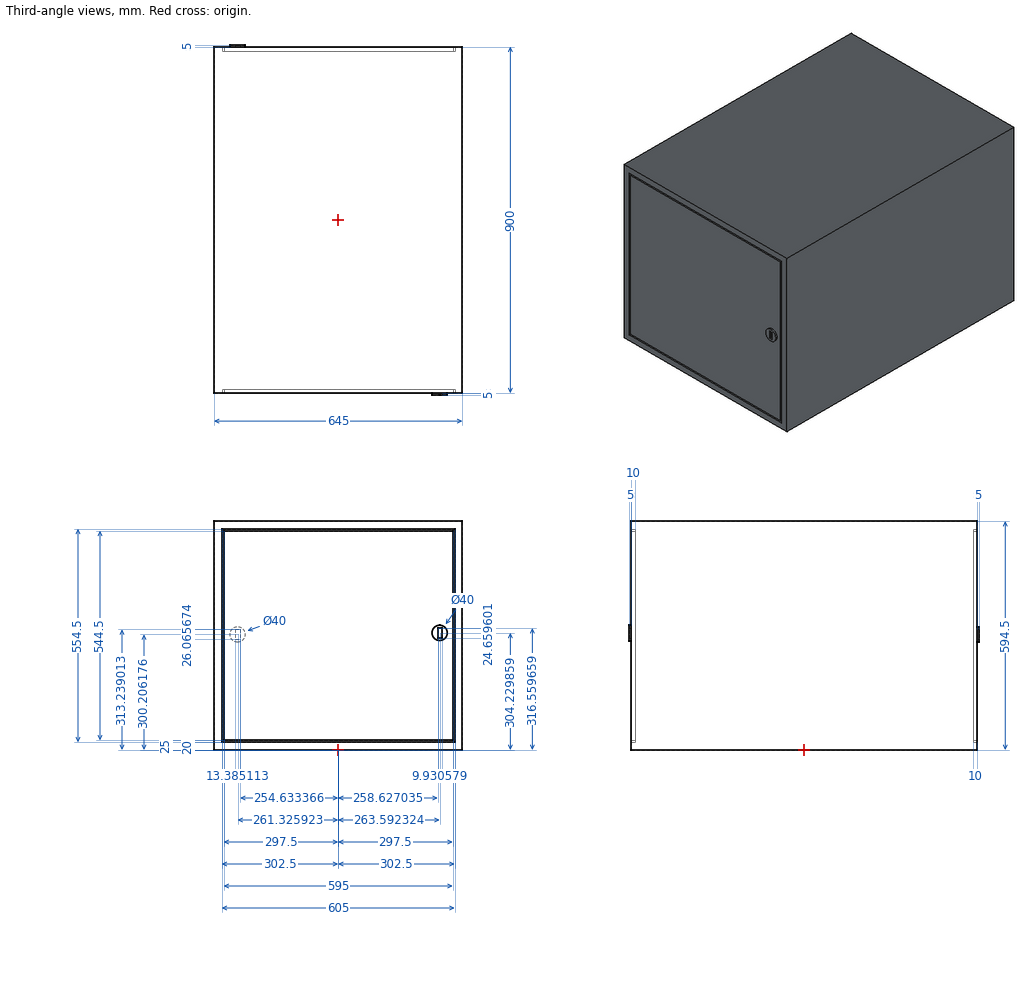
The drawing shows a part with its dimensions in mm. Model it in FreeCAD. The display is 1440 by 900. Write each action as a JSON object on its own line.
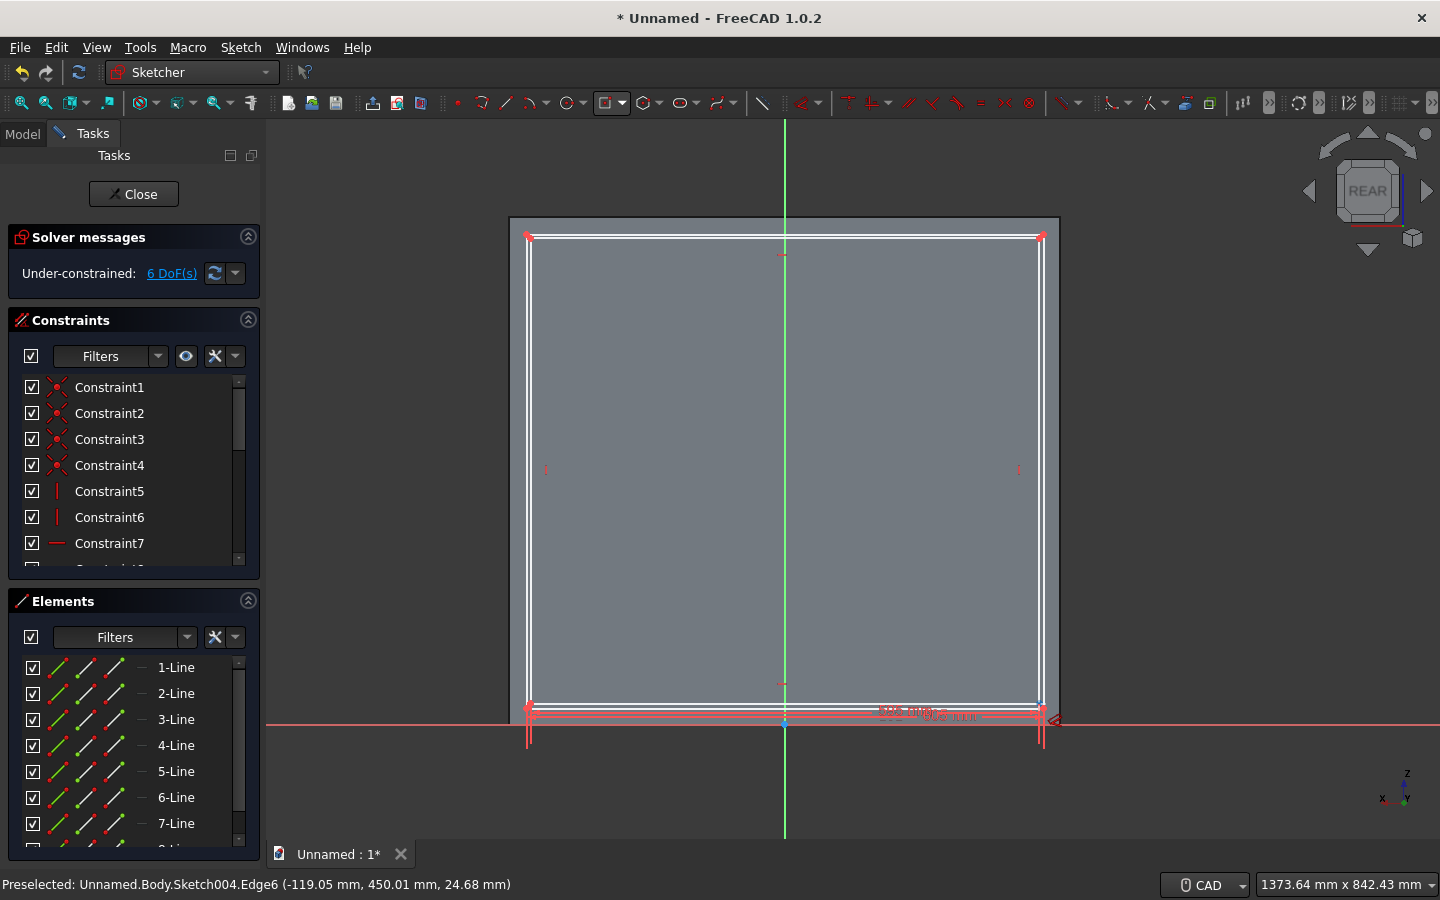
{"action": "scroll", "coordinate": [527, 709], "scroll_direction": "up", "scroll_amount": 5}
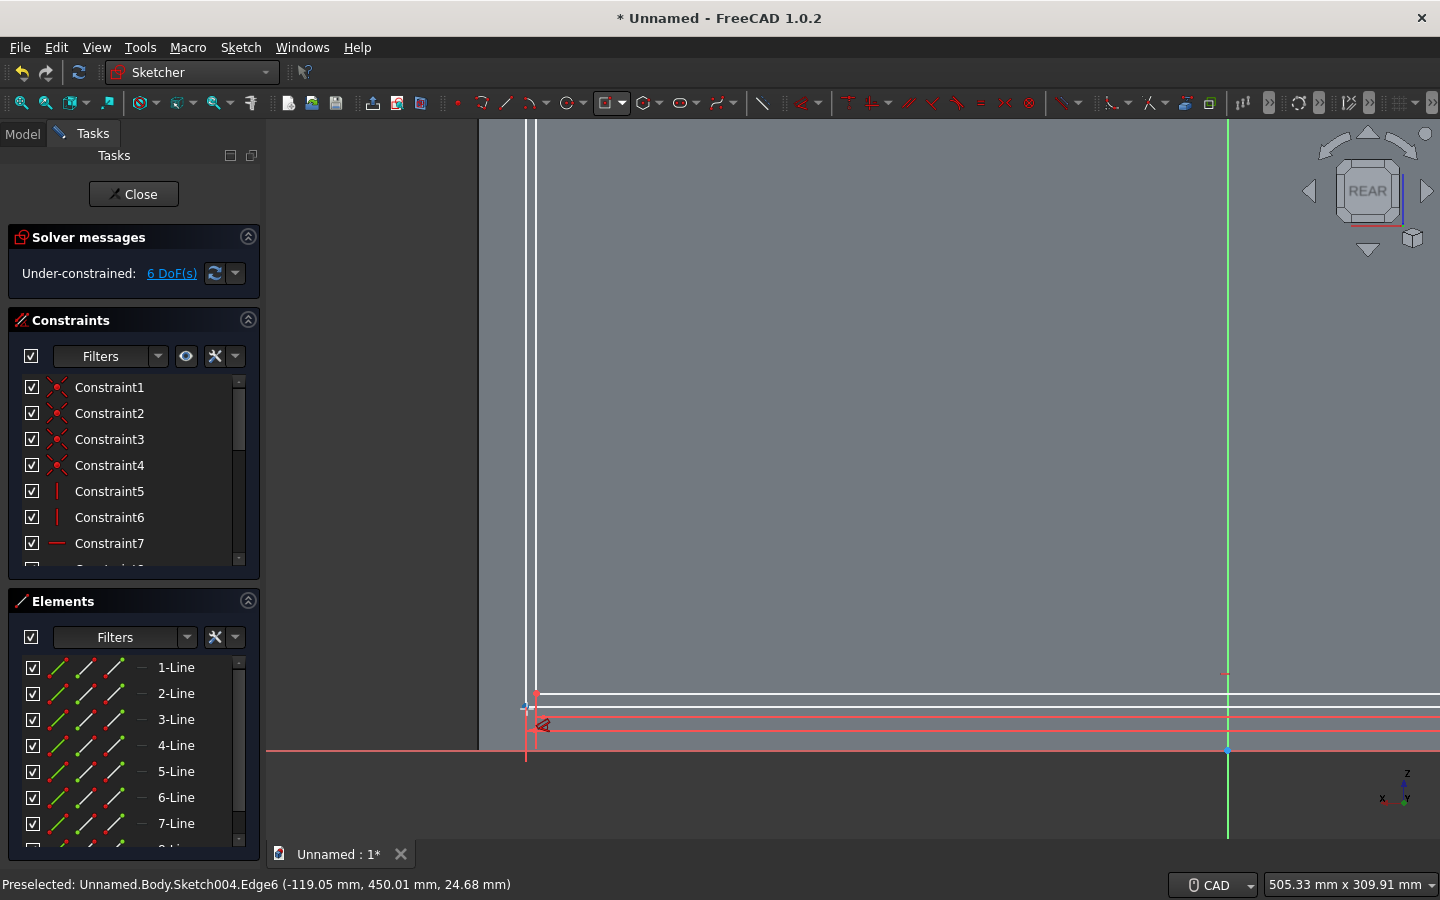
{"action": "left_click", "coordinate": [526, 707]}
{"action": "left_click", "coordinate": [492, 729]}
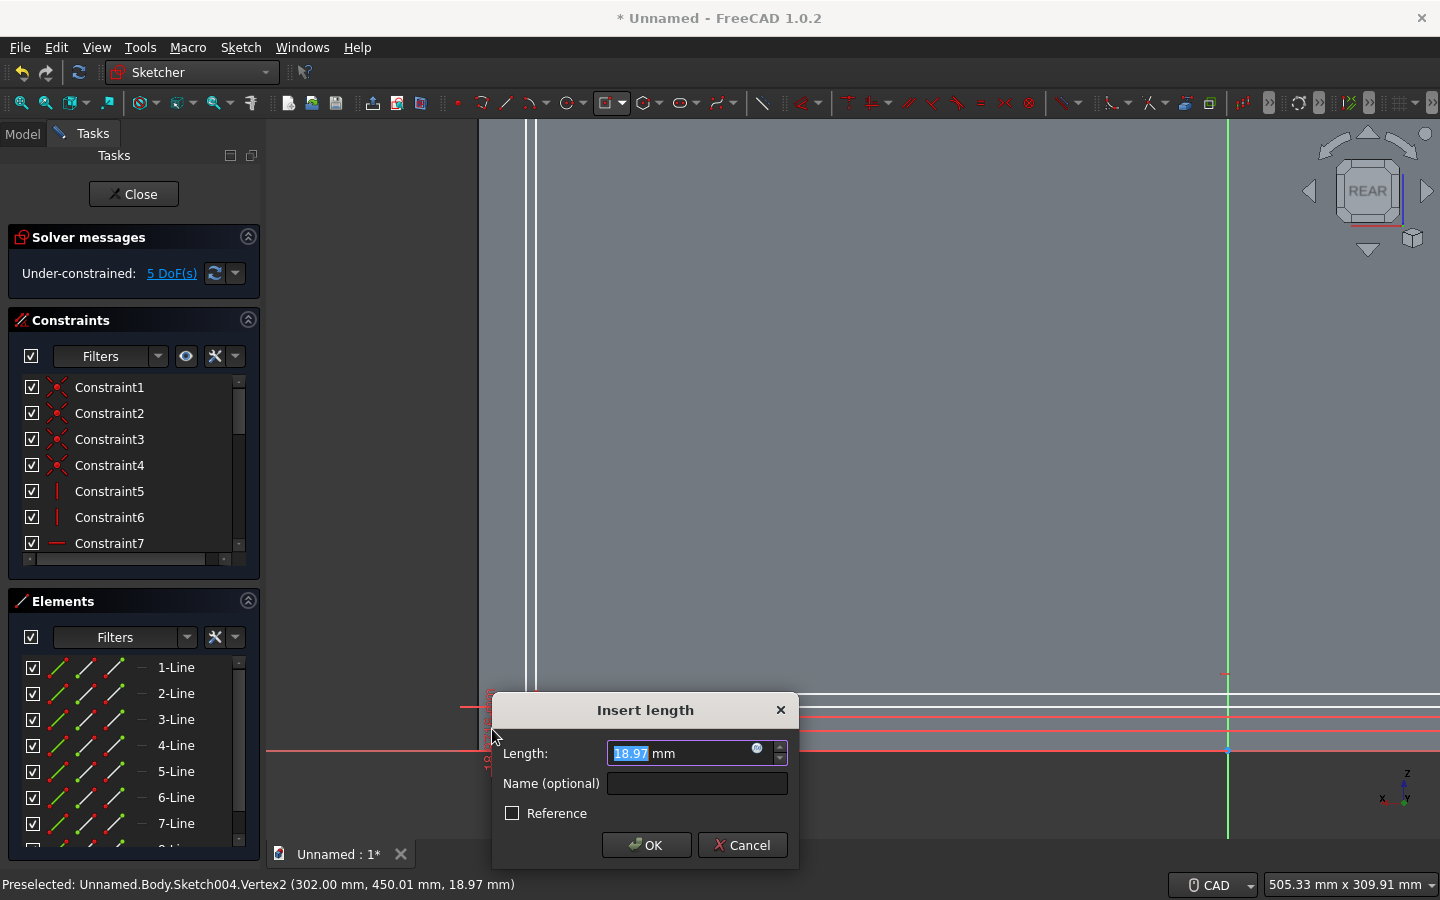
{"action": "type", "text": "20"}
{"action": "key", "text": "Return"}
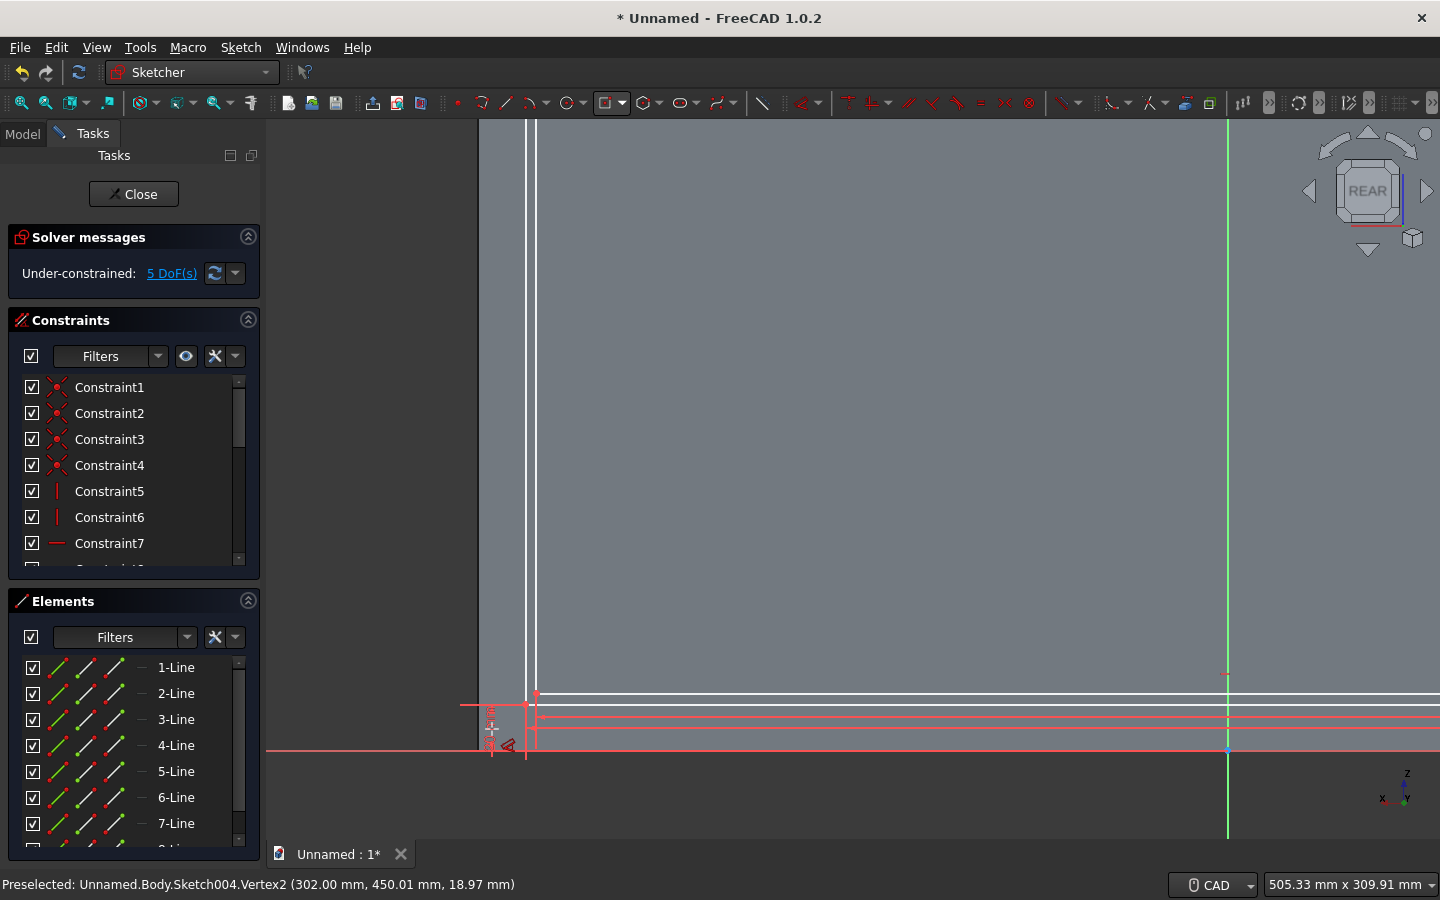
{"action": "left_click", "coordinate": [536, 694]}
{"action": "left_click", "coordinate": [502, 702]}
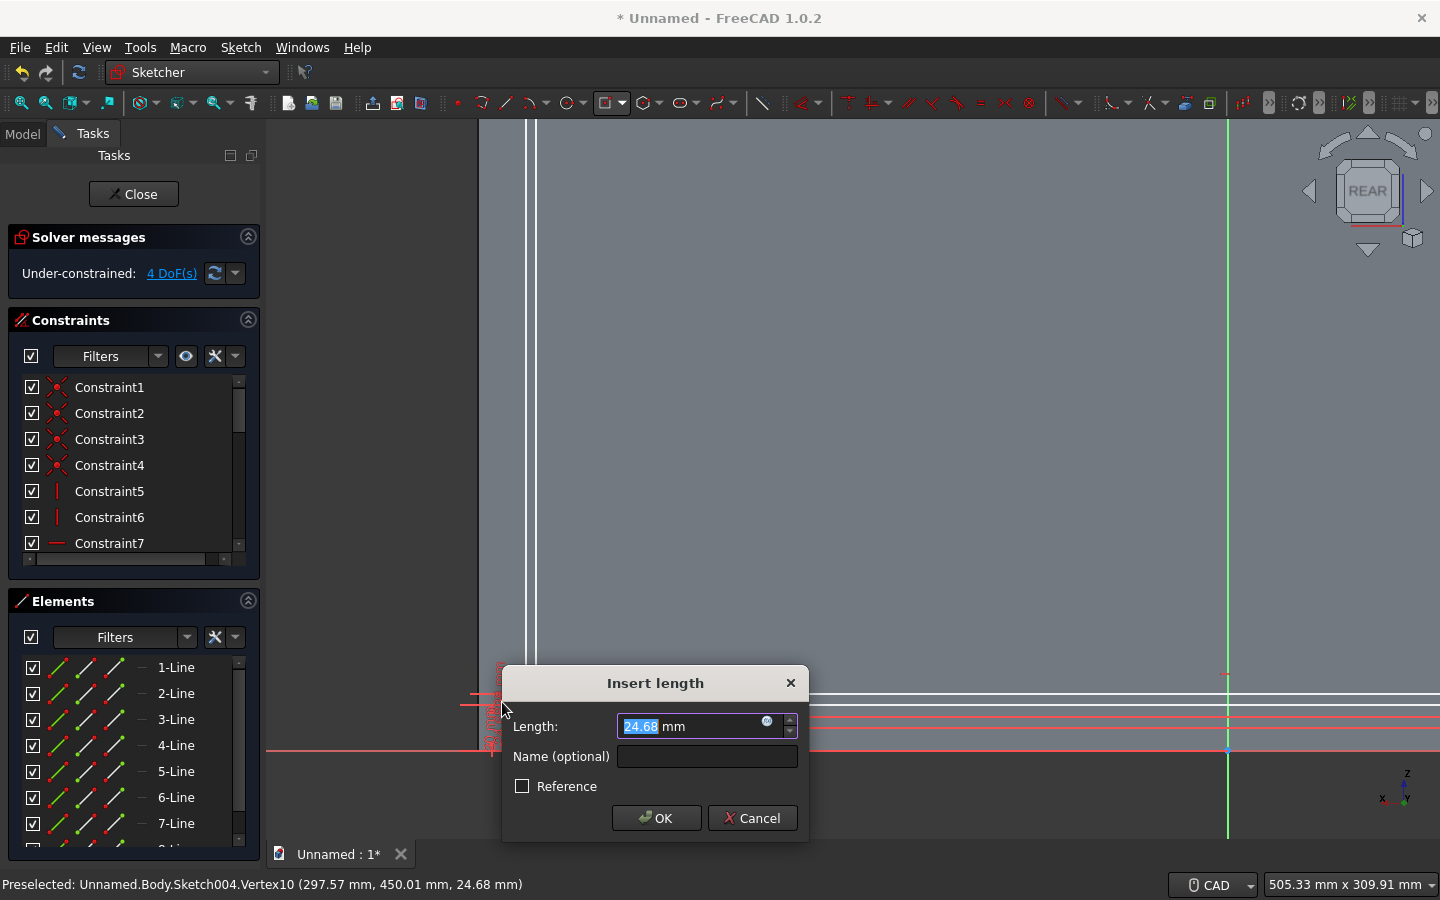
{"action": "type", "text": "25"}
{"action": "key", "text": "Return"}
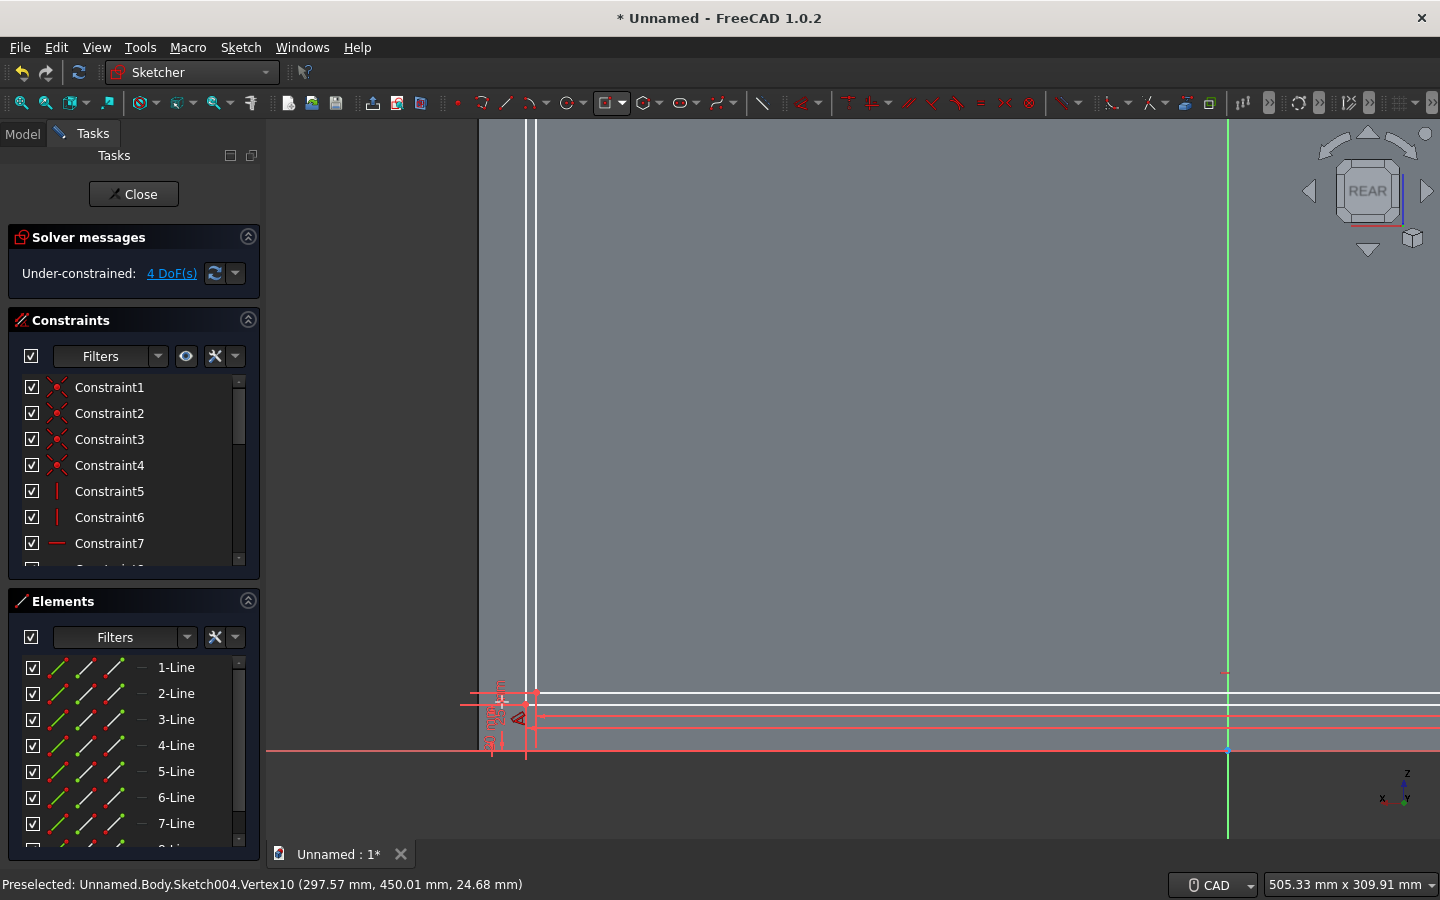
{"action": "scroll", "coordinate": [526, 319], "scroll_direction": "up", "scroll_amount": 2}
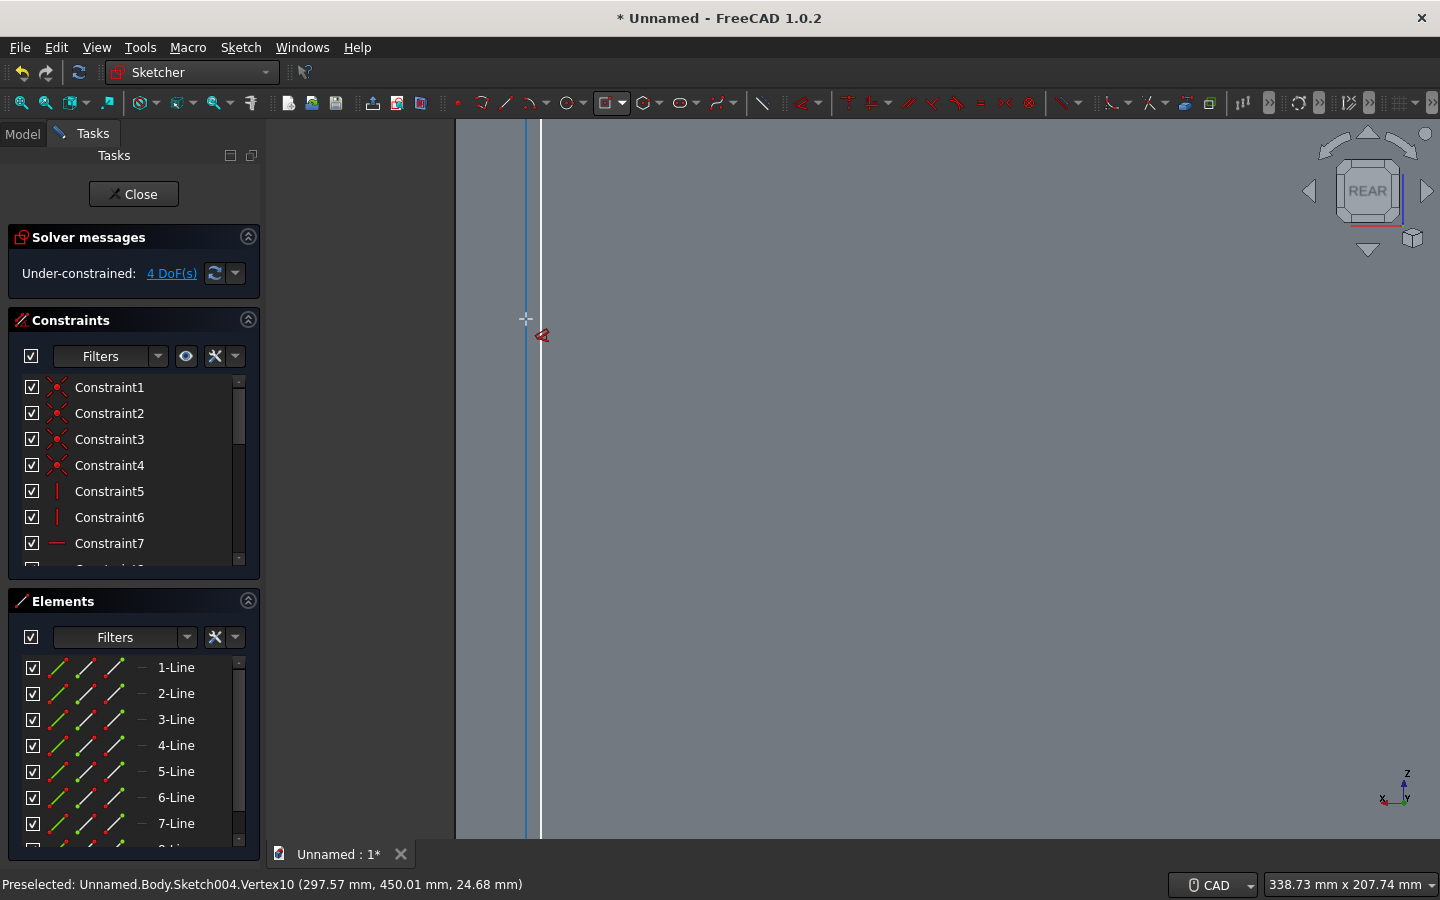
{"action": "left_click", "coordinate": [526, 318]}
{"action": "left_click", "coordinate": [492, 479]}